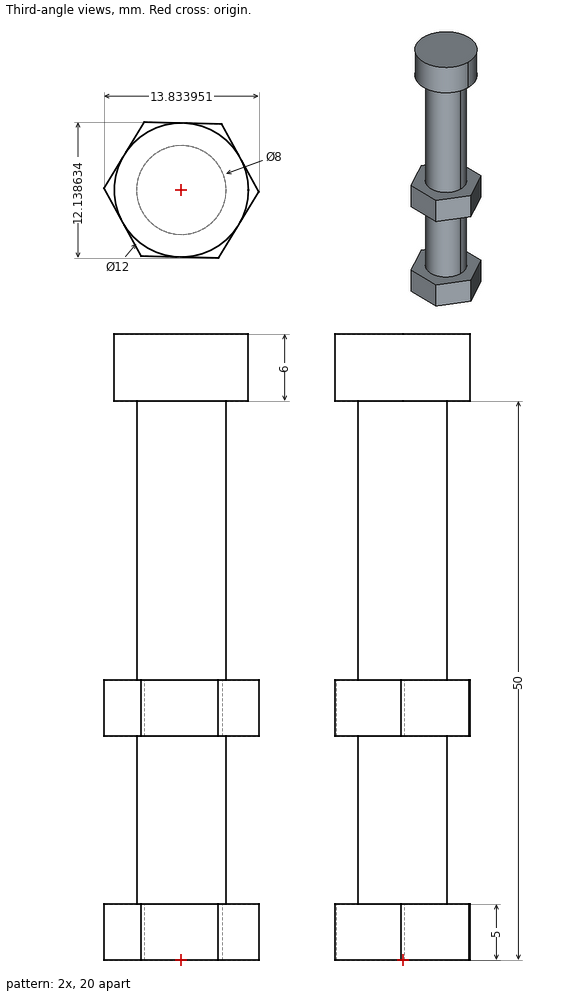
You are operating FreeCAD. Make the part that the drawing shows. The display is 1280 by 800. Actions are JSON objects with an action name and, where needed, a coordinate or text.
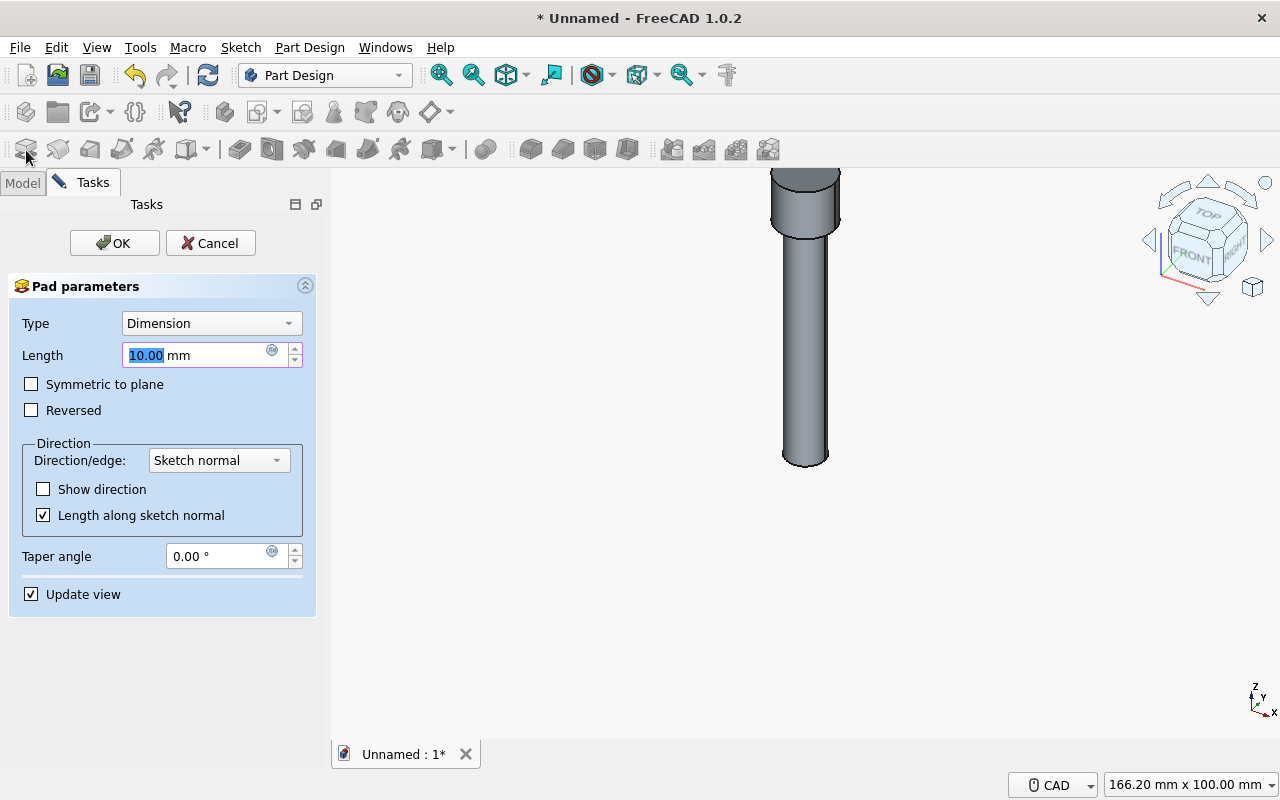
{"action": "type", "text": "6"}
{"action": "key", "text": "Tab"}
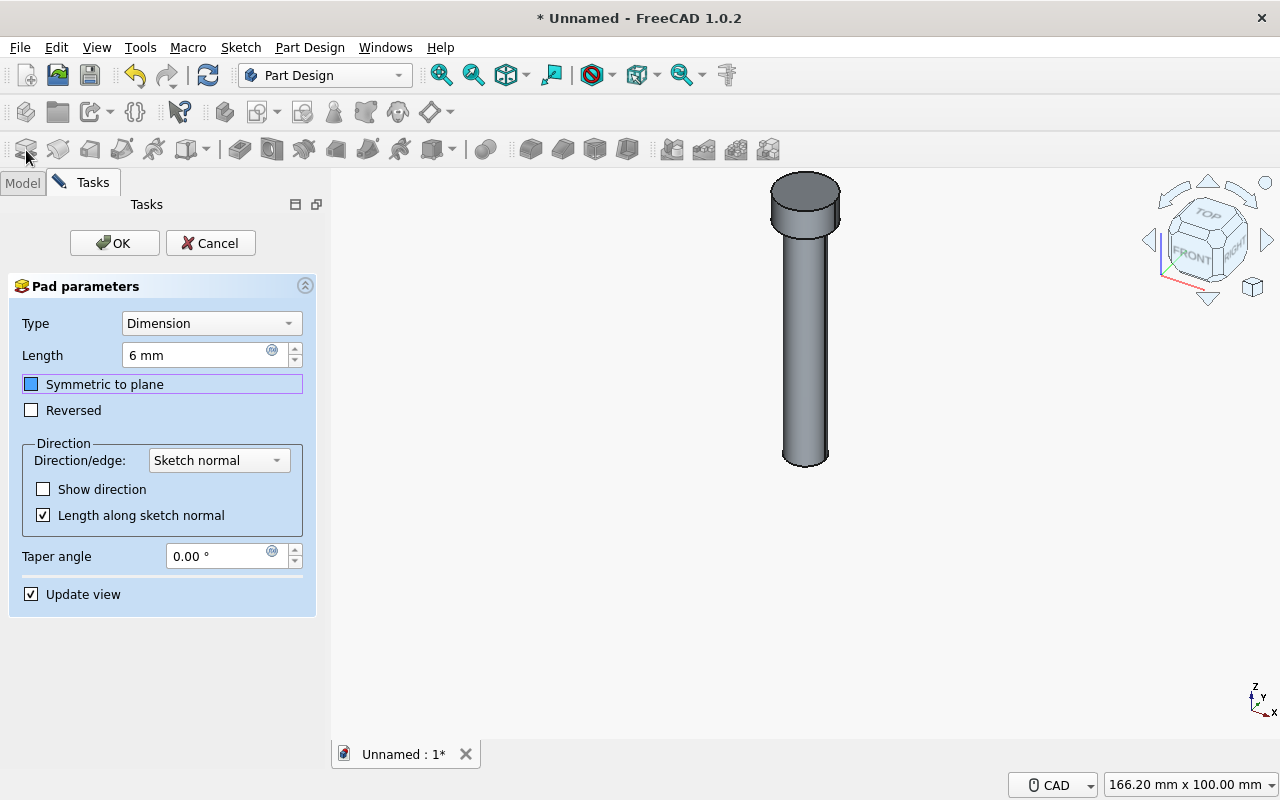
{"action": "left_click", "coordinate": [115, 243]}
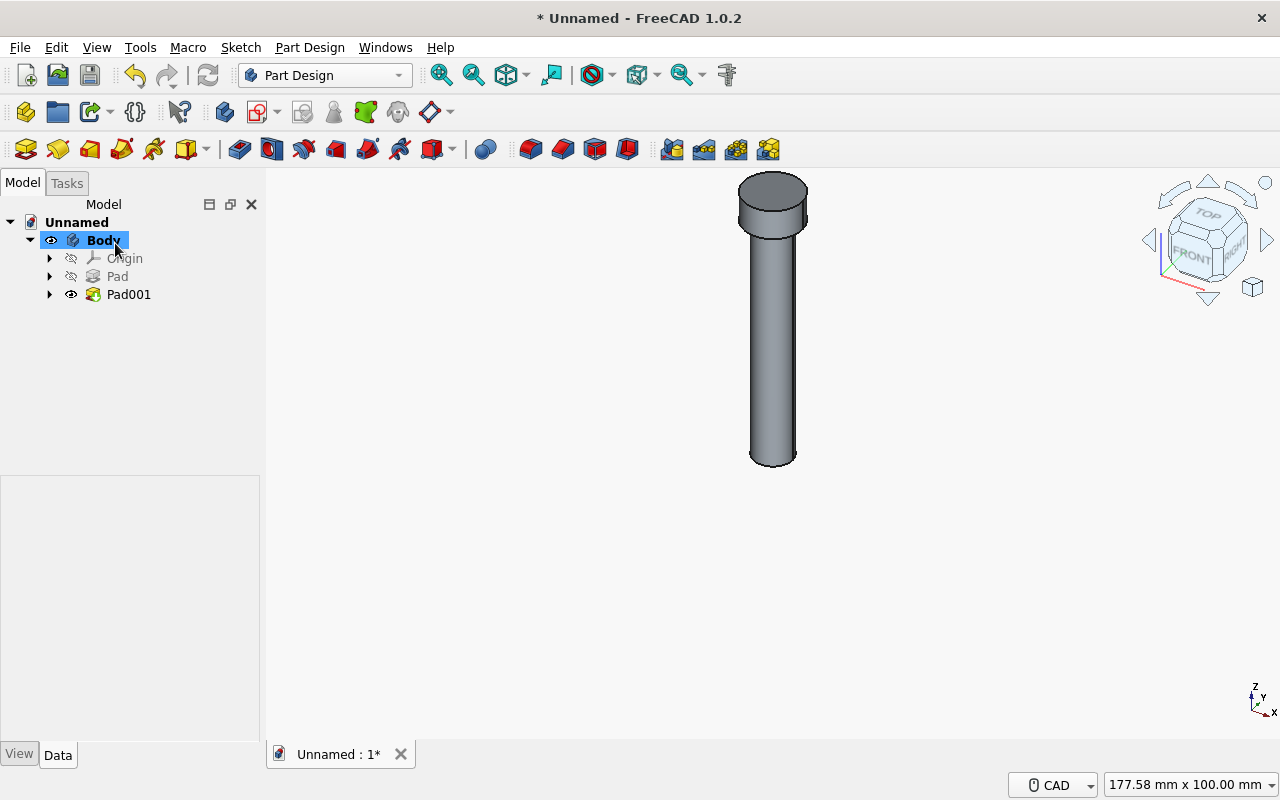
{"action": "left_click", "coordinate": [442, 76]}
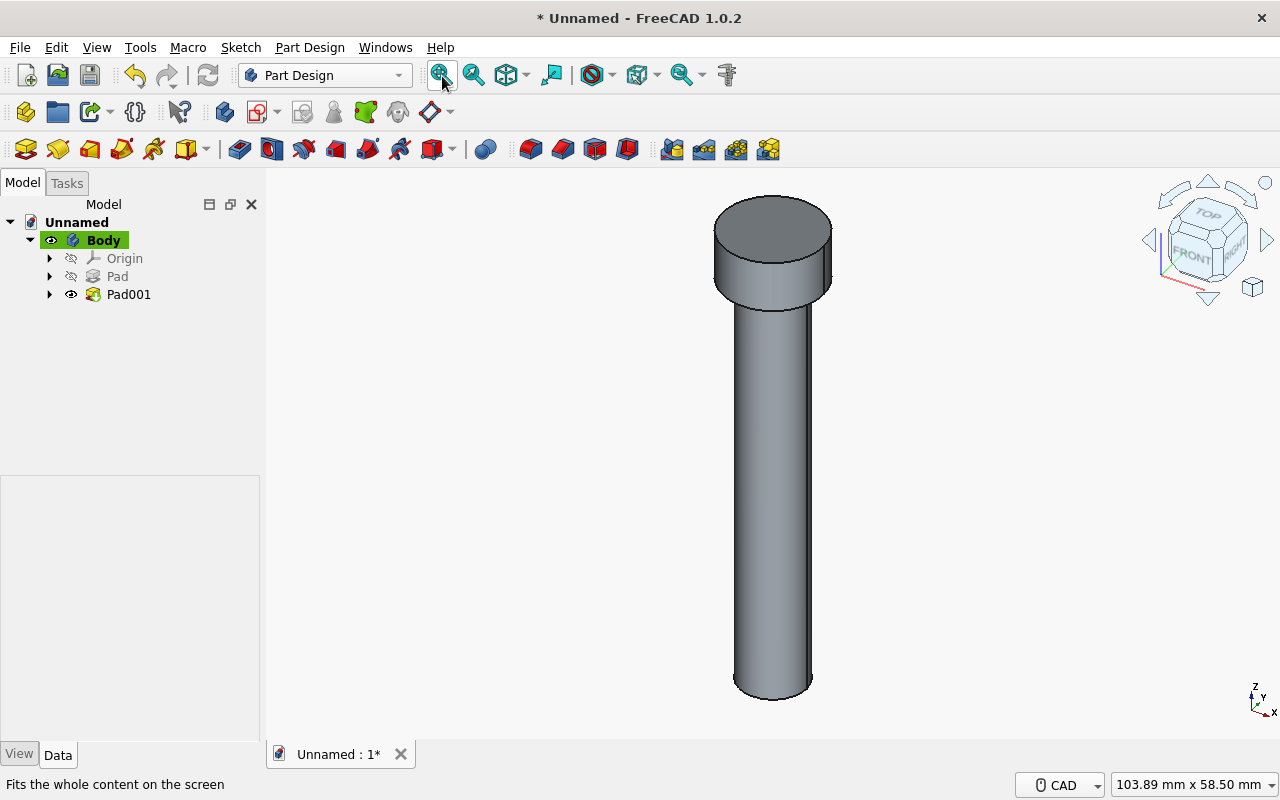
{"action": "key", "text": "5"}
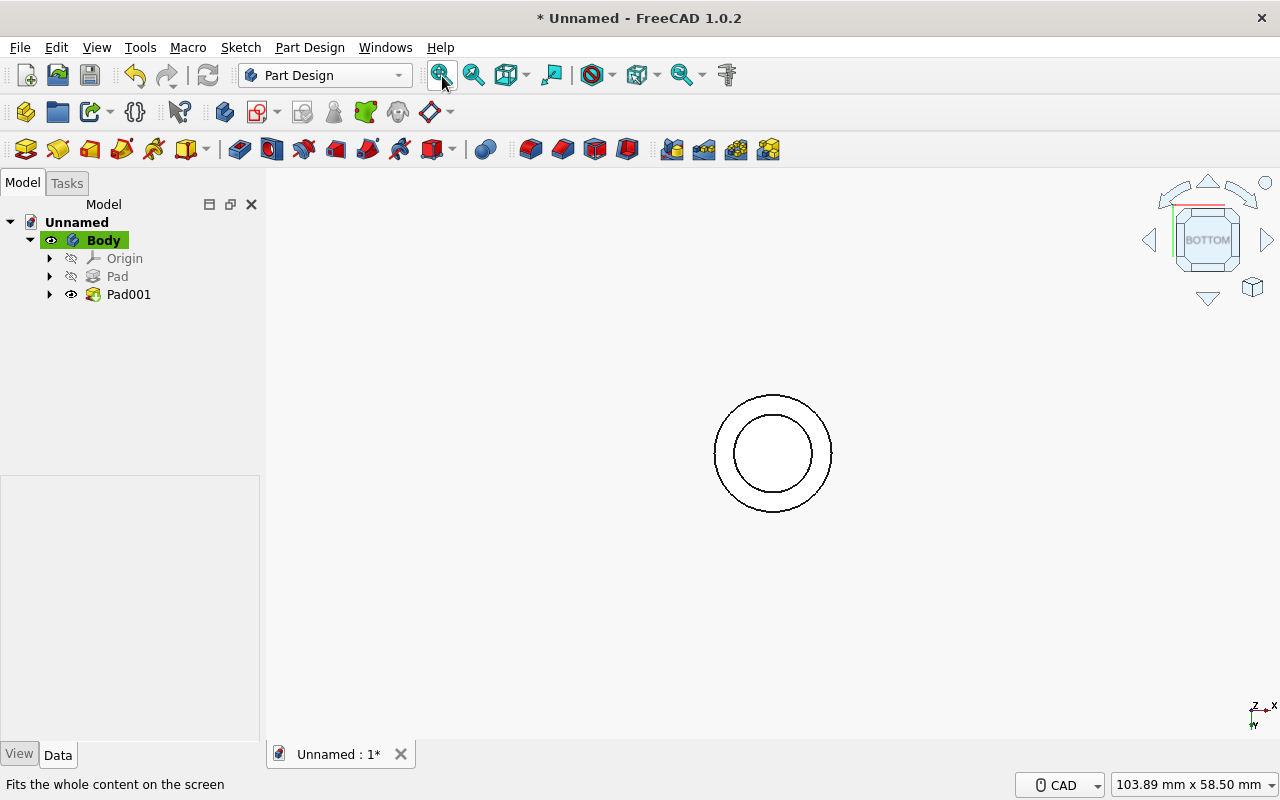
{"action": "left_click", "coordinate": [442, 76]}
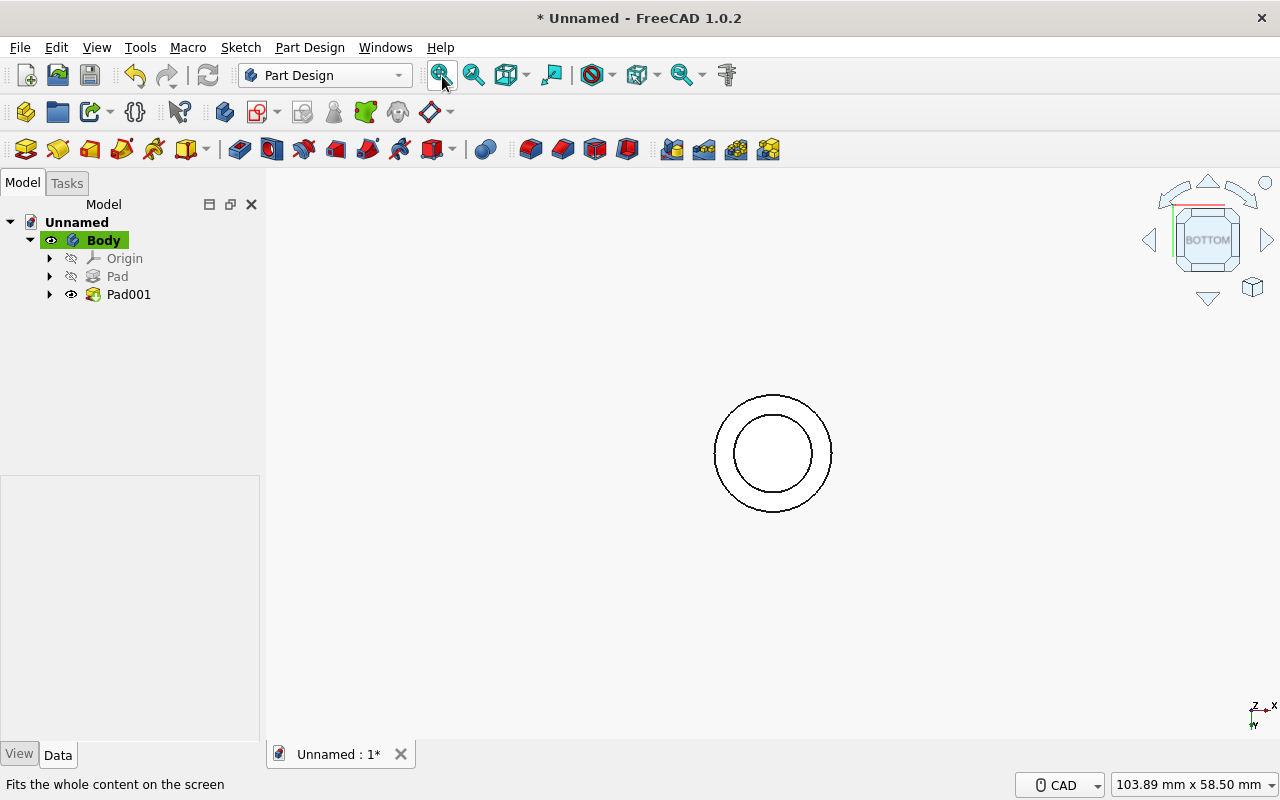
{"action": "left_click", "coordinate": [773, 452]}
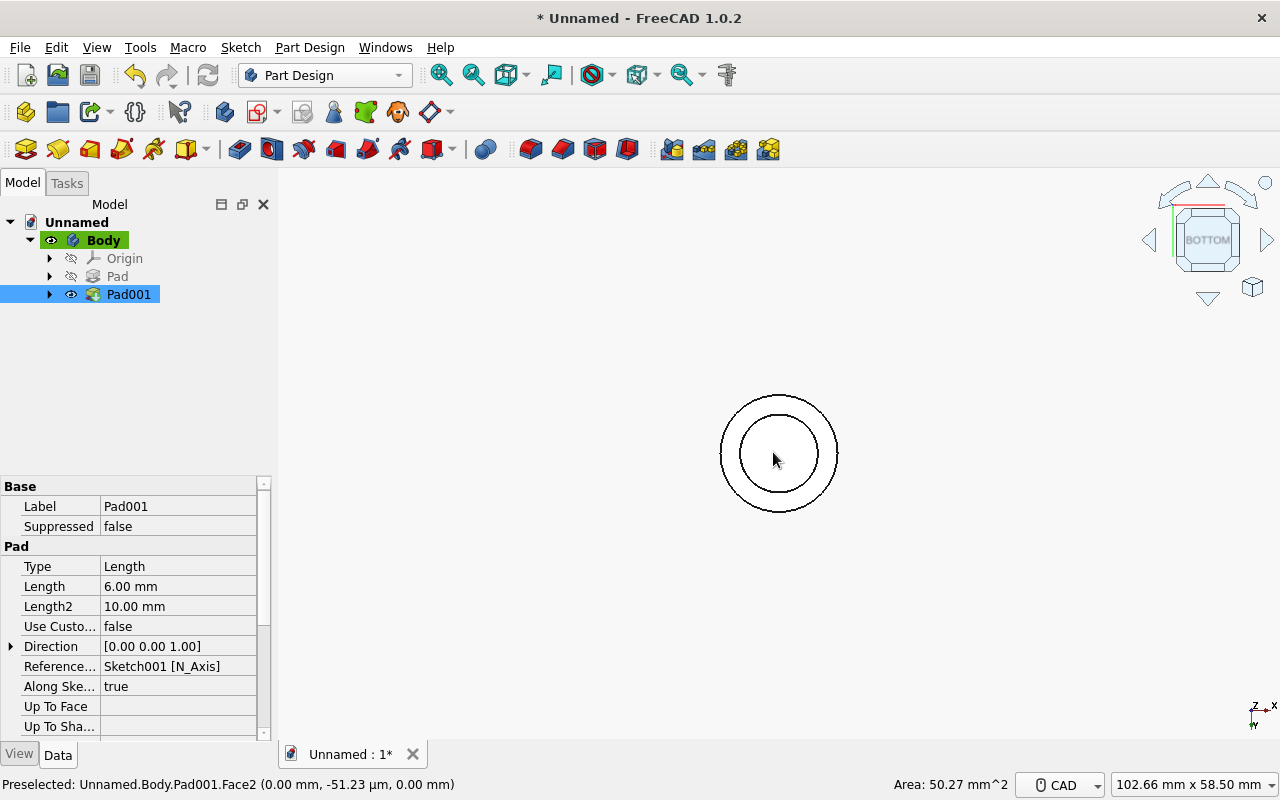
{"action": "left_click", "coordinate": [258, 112]}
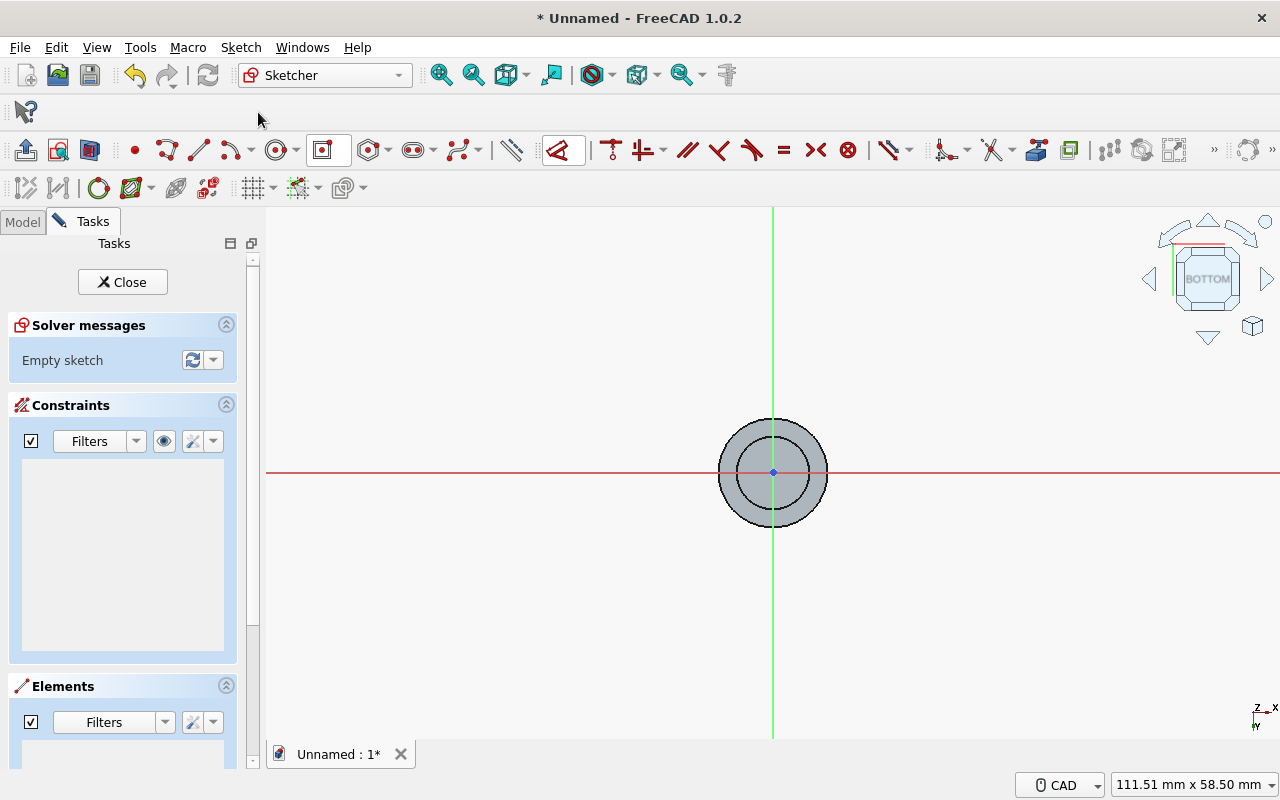
{"action": "scroll", "coordinate": [803, 473], "scroll_direction": "up", "scroll_amount": 6}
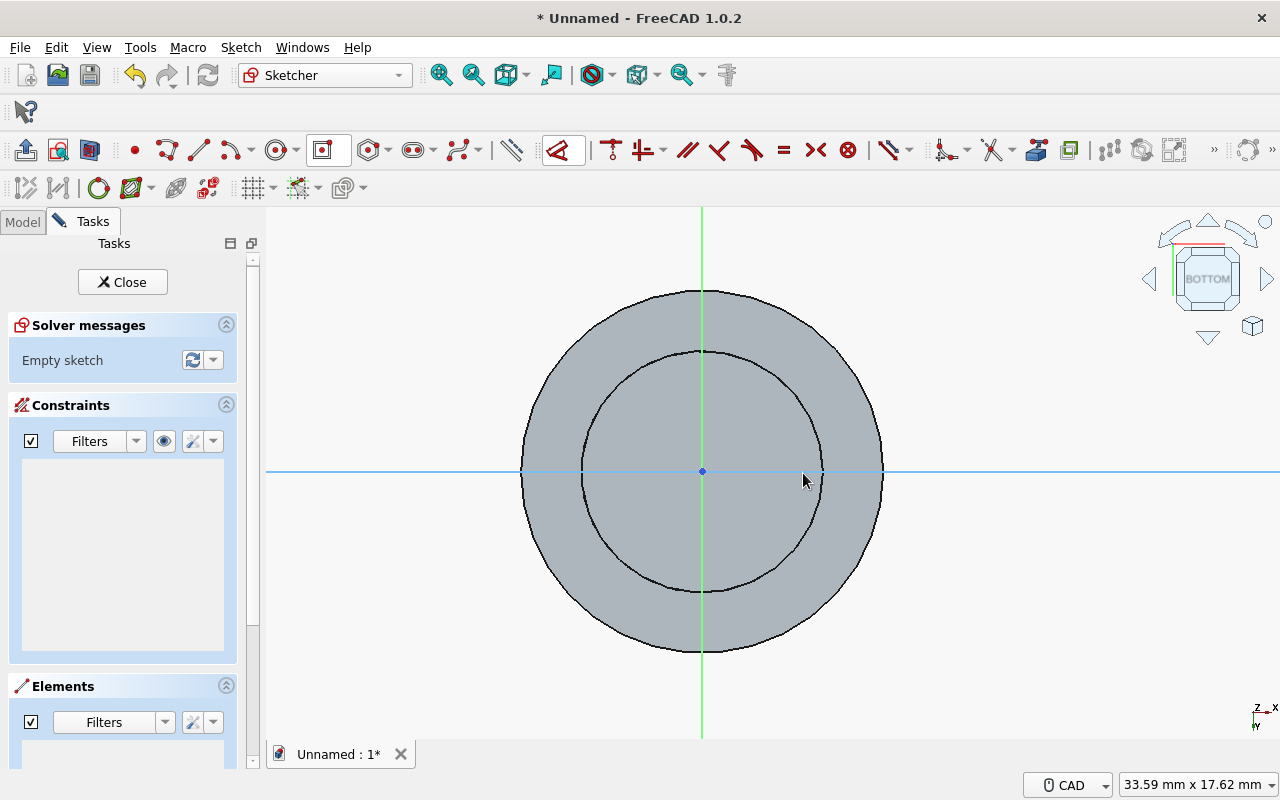
{"action": "left_click", "coordinate": [368, 150]}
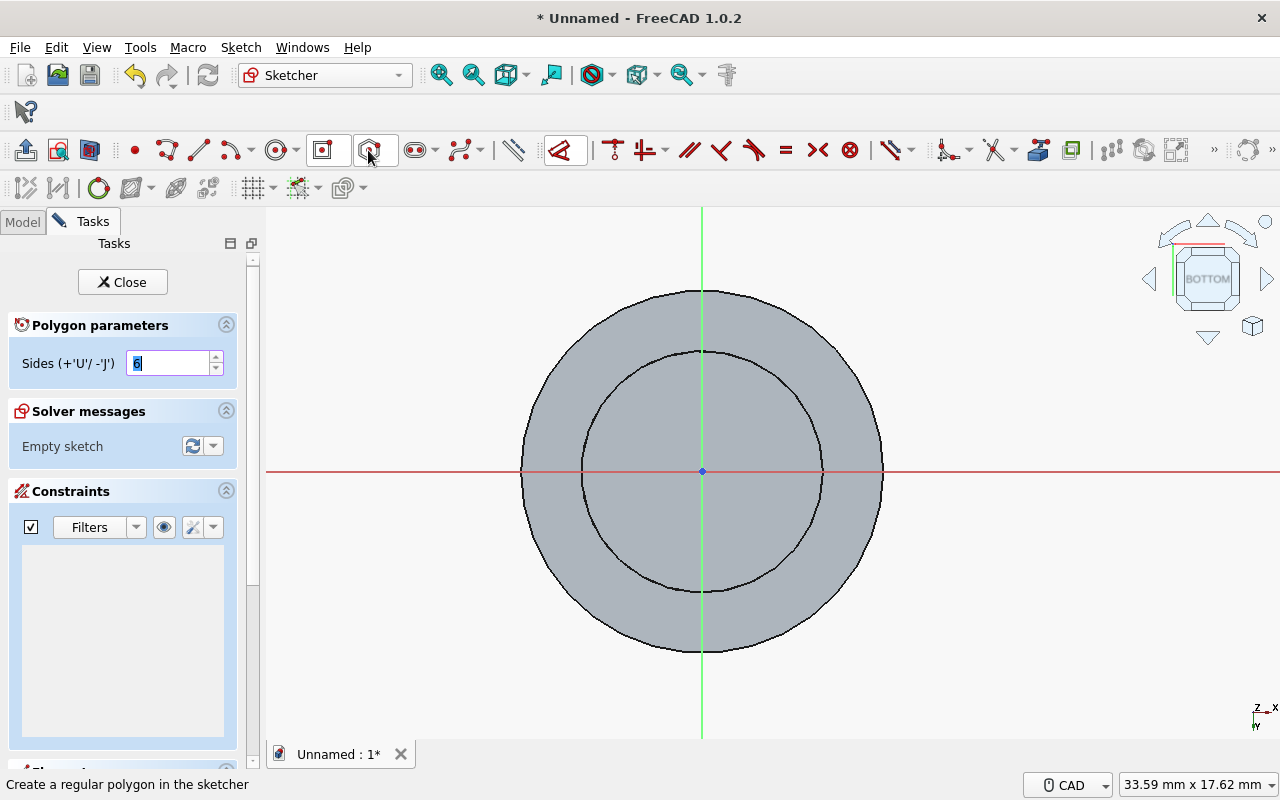
{"action": "left_click", "coordinate": [702, 472]}